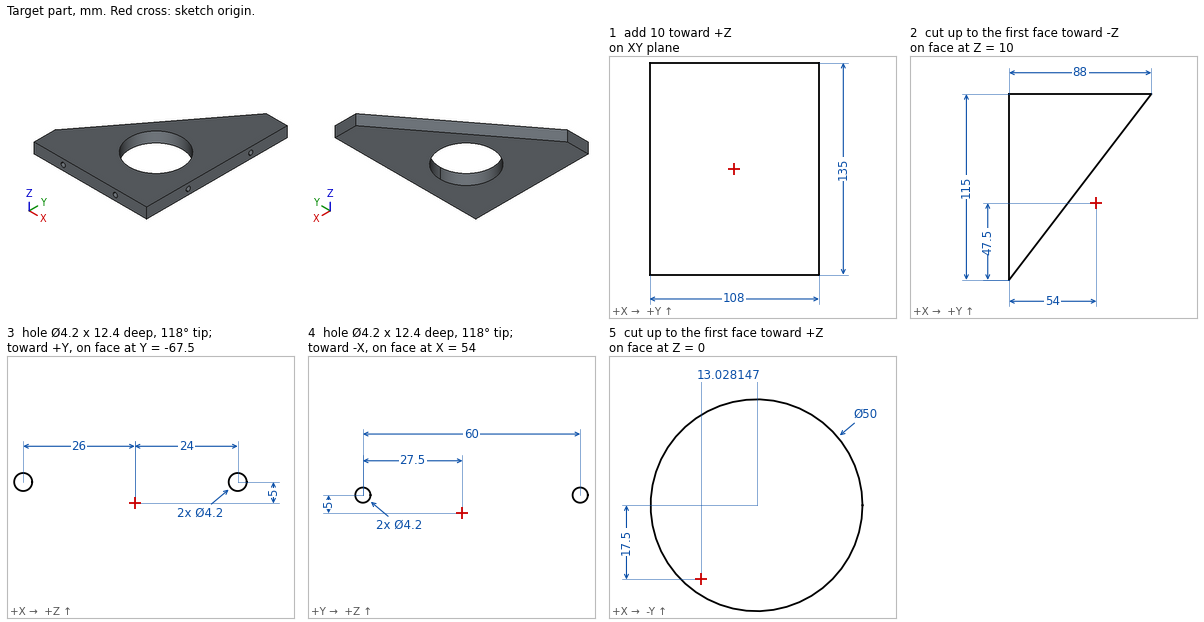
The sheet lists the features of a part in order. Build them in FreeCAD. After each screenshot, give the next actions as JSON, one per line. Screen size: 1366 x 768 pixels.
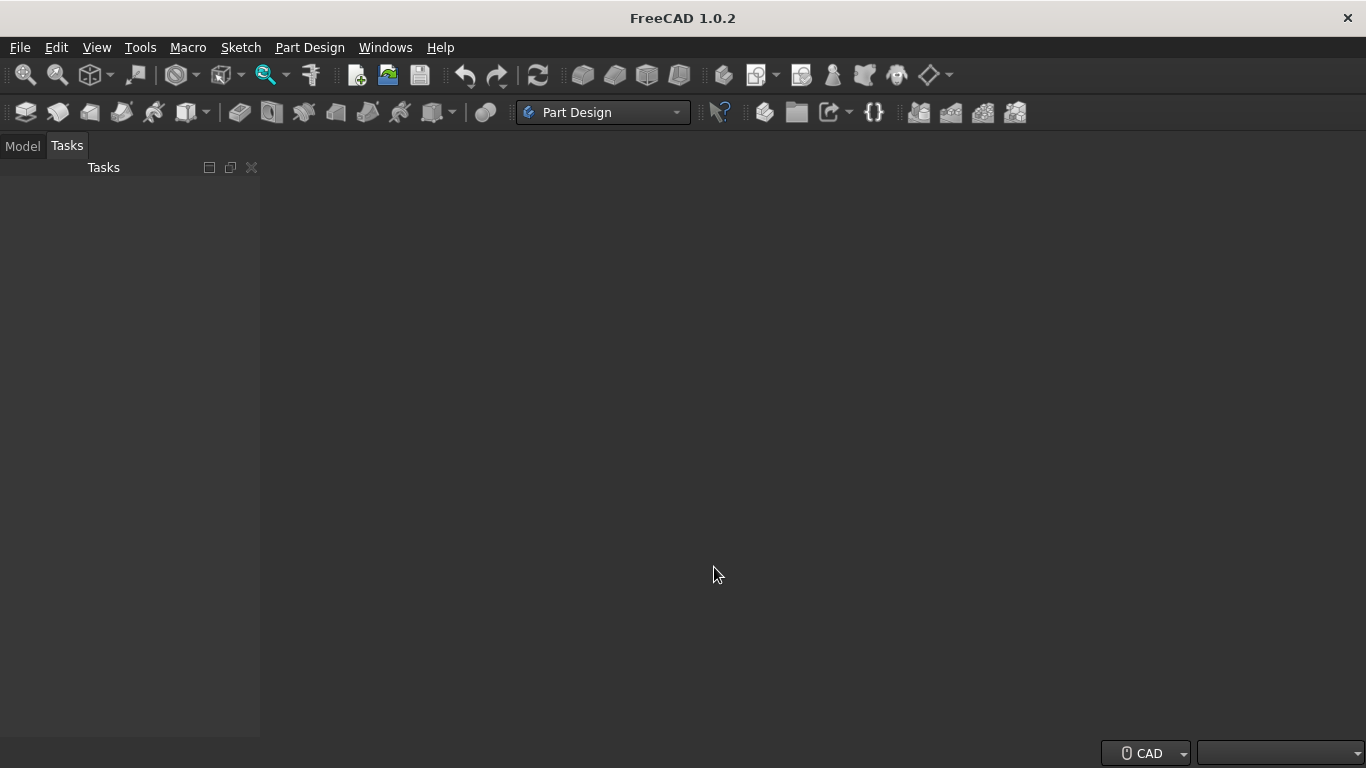
{"action": "key", "text": "ctrl+n"}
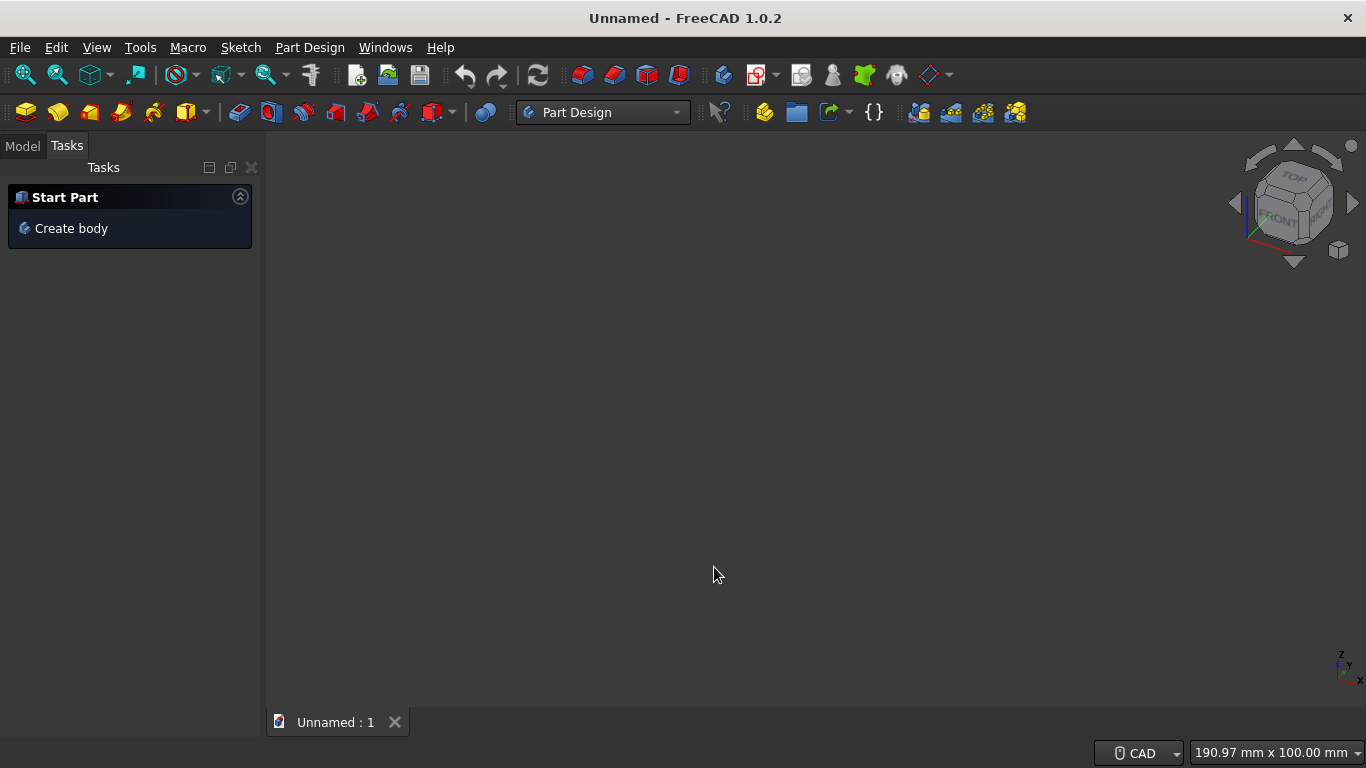
{"action": "left_click", "coordinate": [756, 76]}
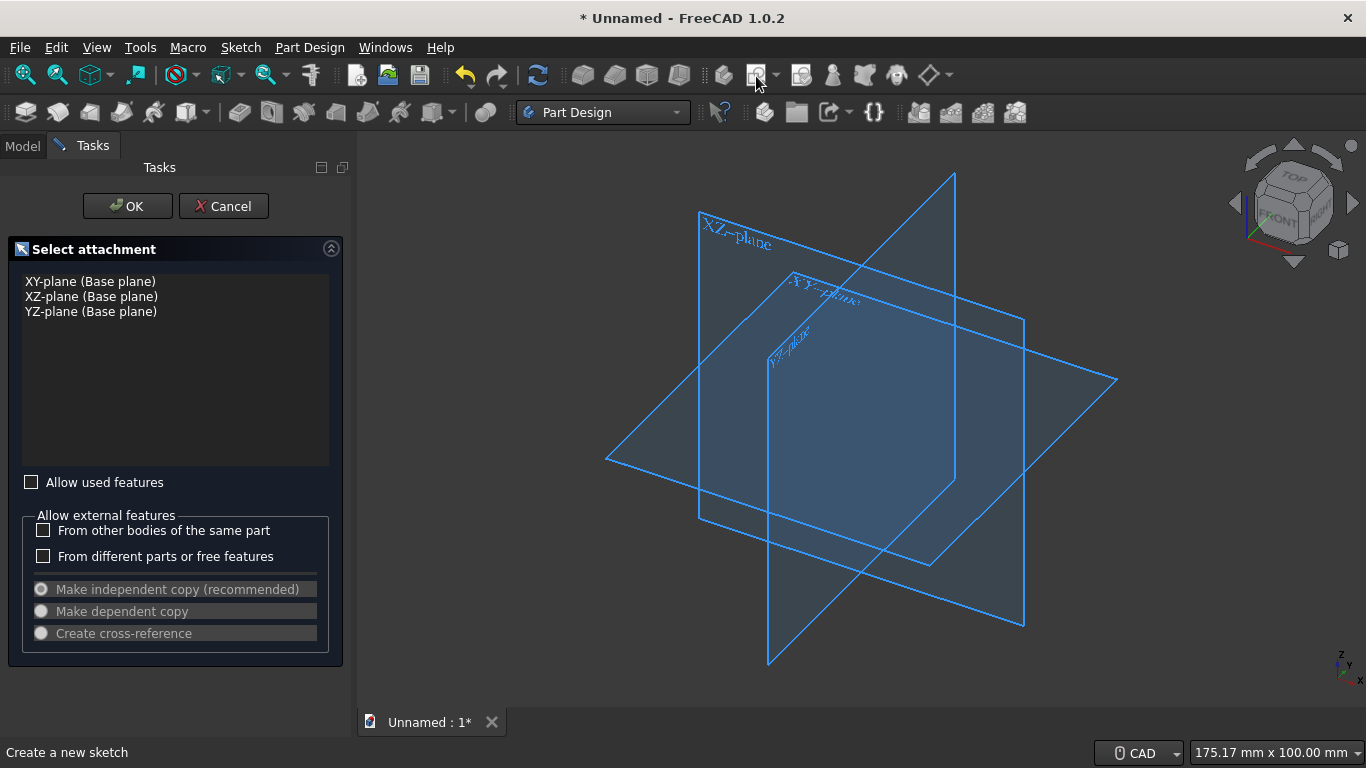
{"action": "left_click", "coordinate": [82, 282]}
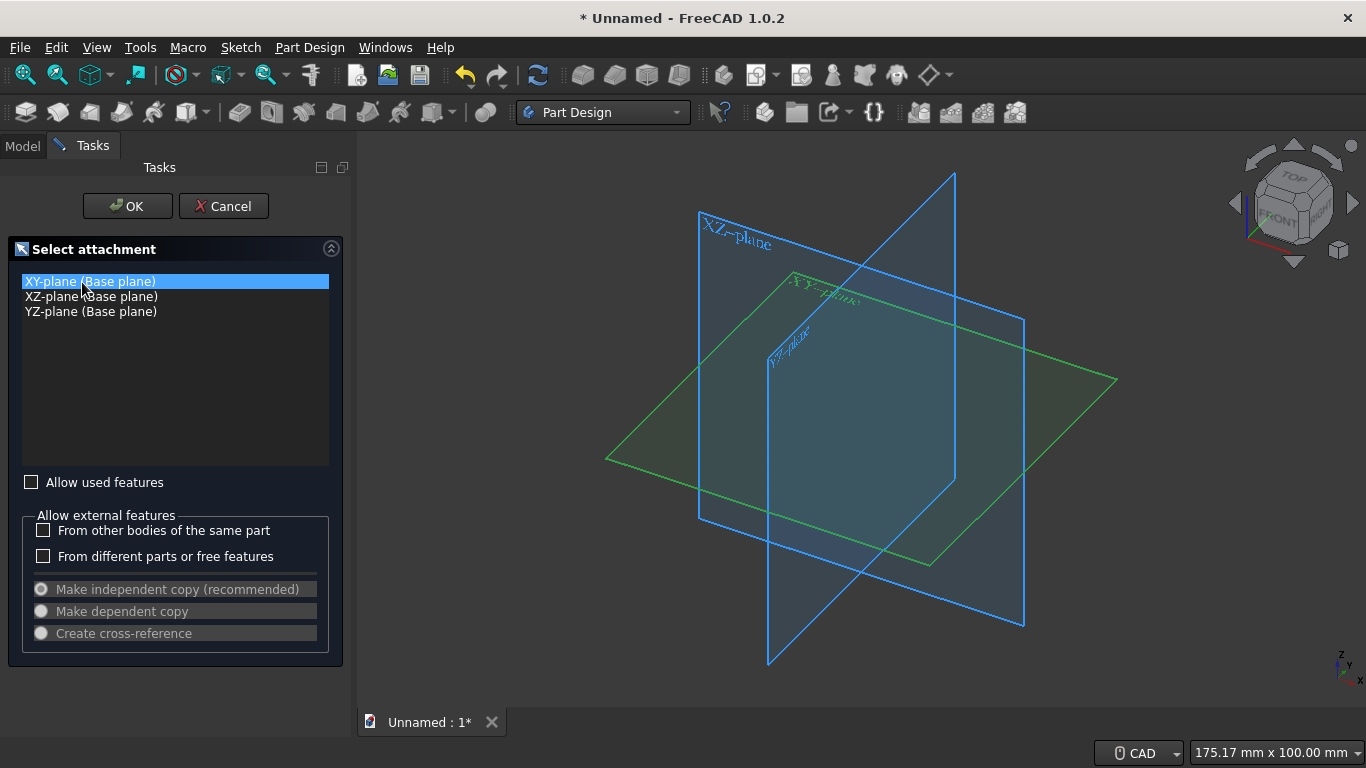
{"action": "left_click", "coordinate": [128, 206]}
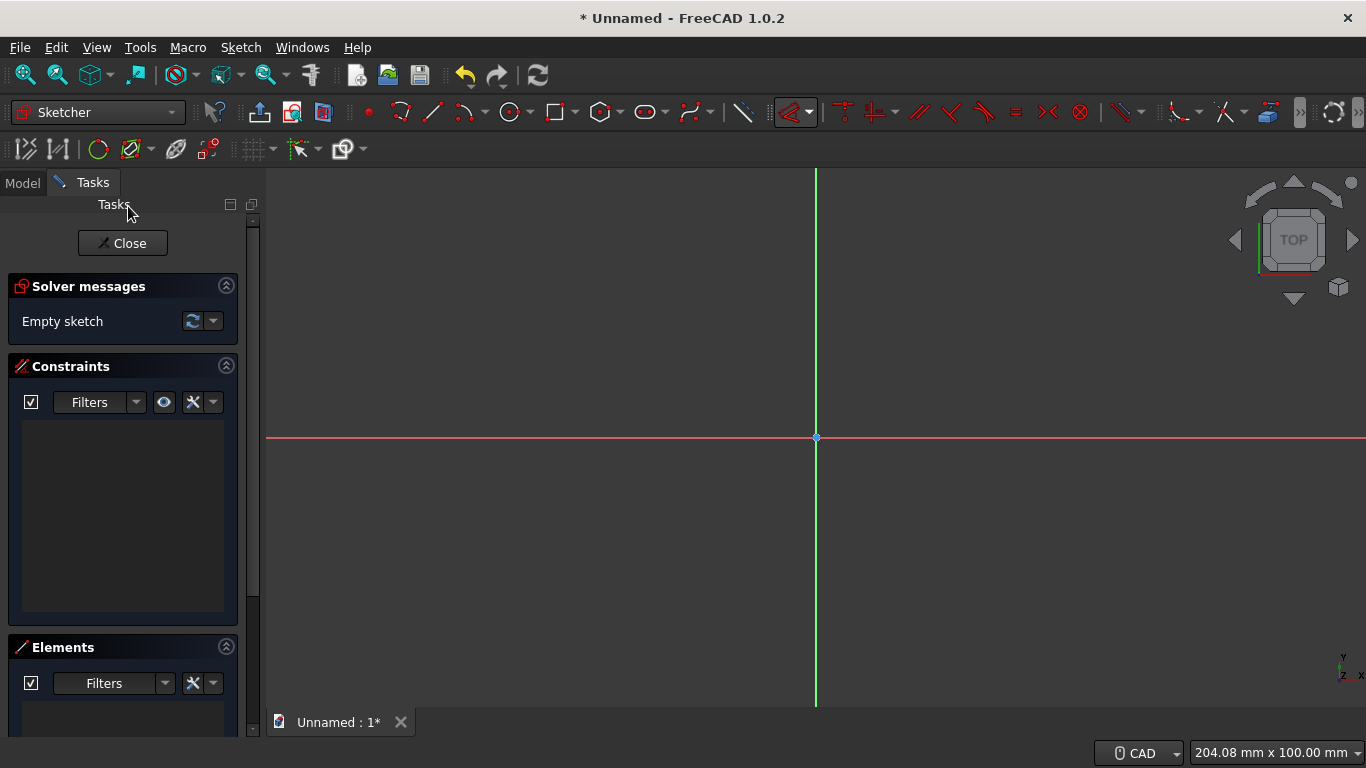
{"action": "scroll", "coordinate": [692, 438], "scroll_direction": "down", "scroll_amount": 4}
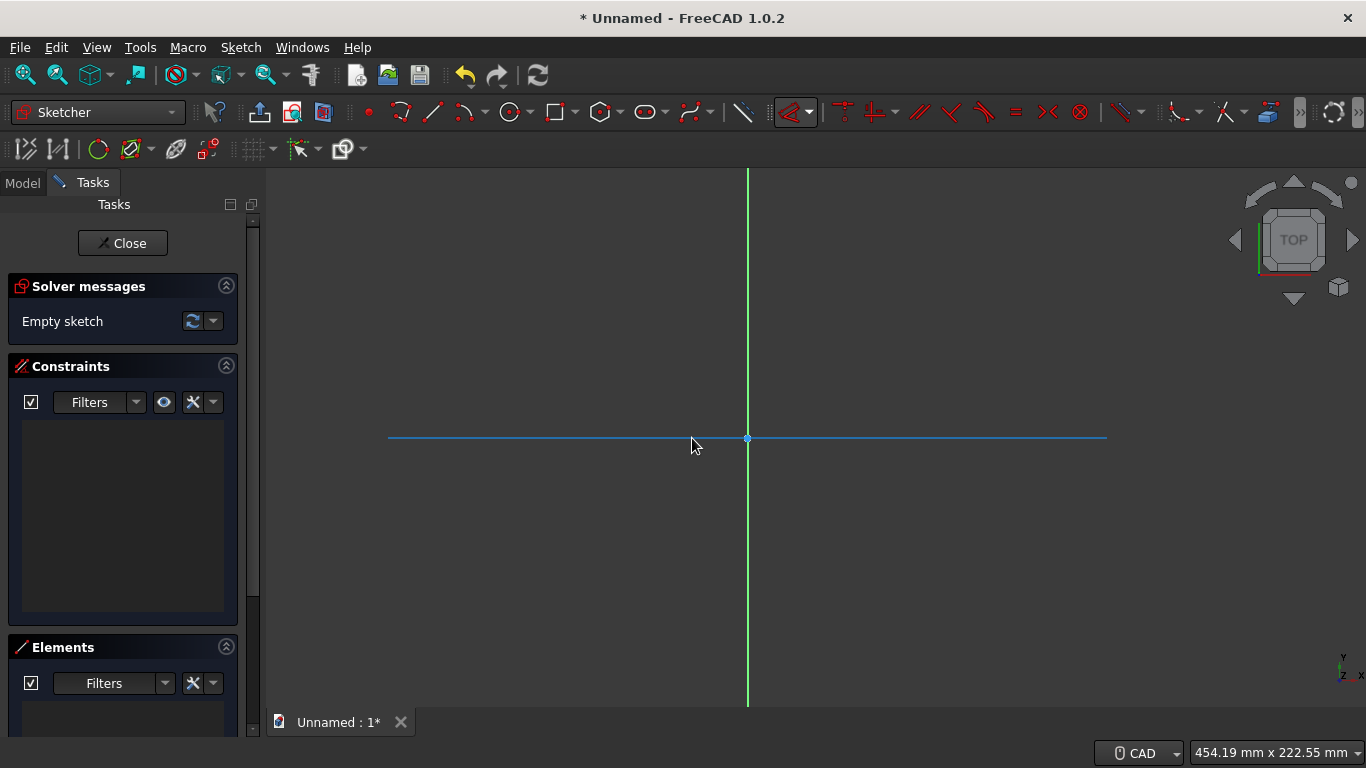
{"action": "key", "text": "g v"}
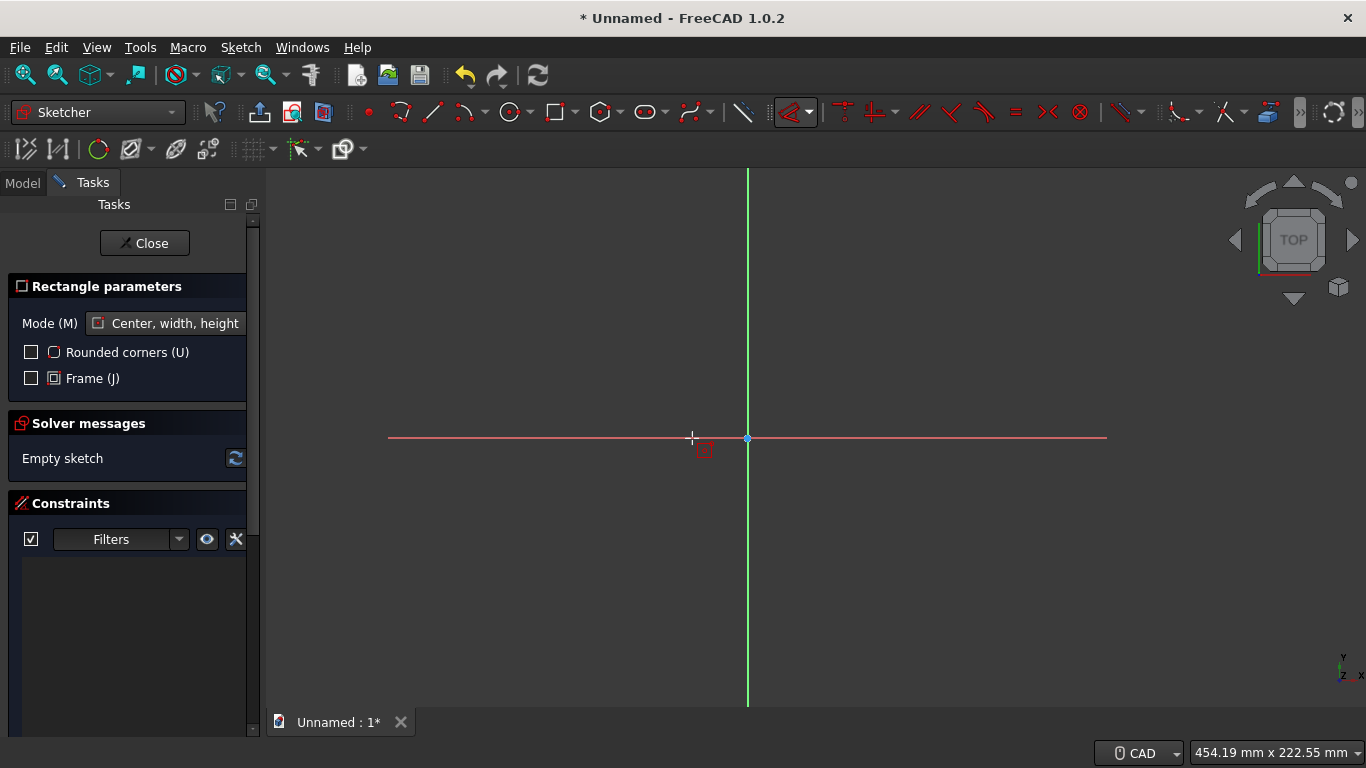
{"action": "left_click", "coordinate": [748, 438]}
{"action": "mouse_move", "coordinate": [879, 275]}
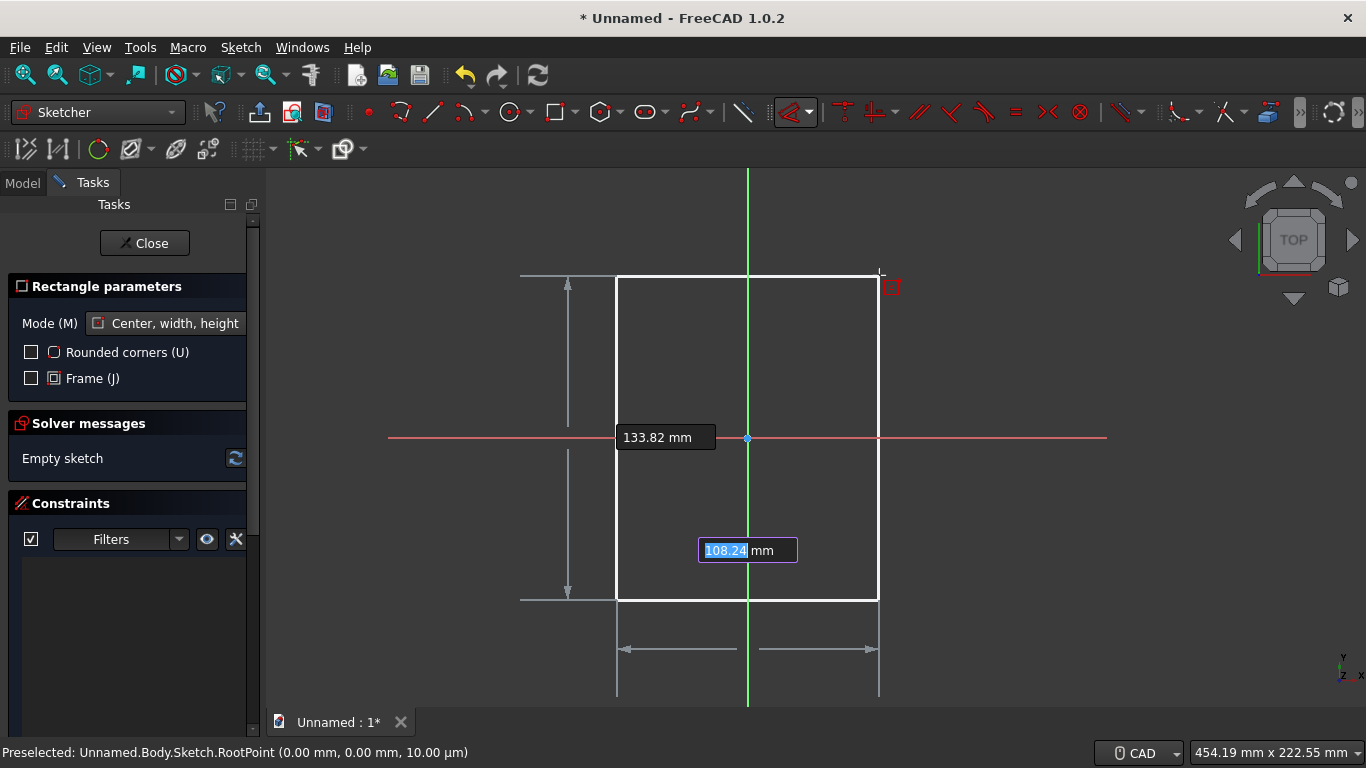
{"action": "type", "text": "108"}
{"action": "key", "text": "Tab"}
{"action": "type", "text": "135"}
{"action": "key", "text": "Return"}
{"action": "key", "text": "Escape"}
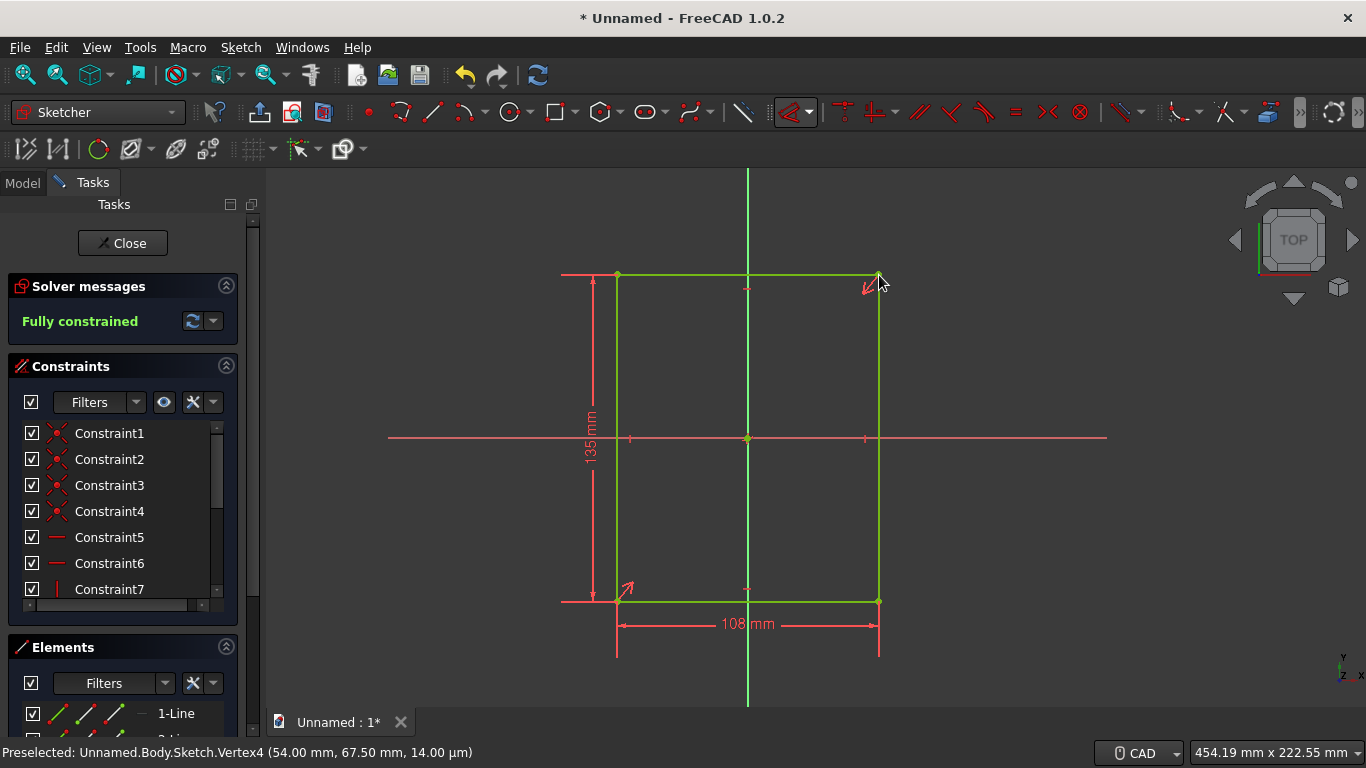
{"action": "left_click", "coordinate": [123, 243]}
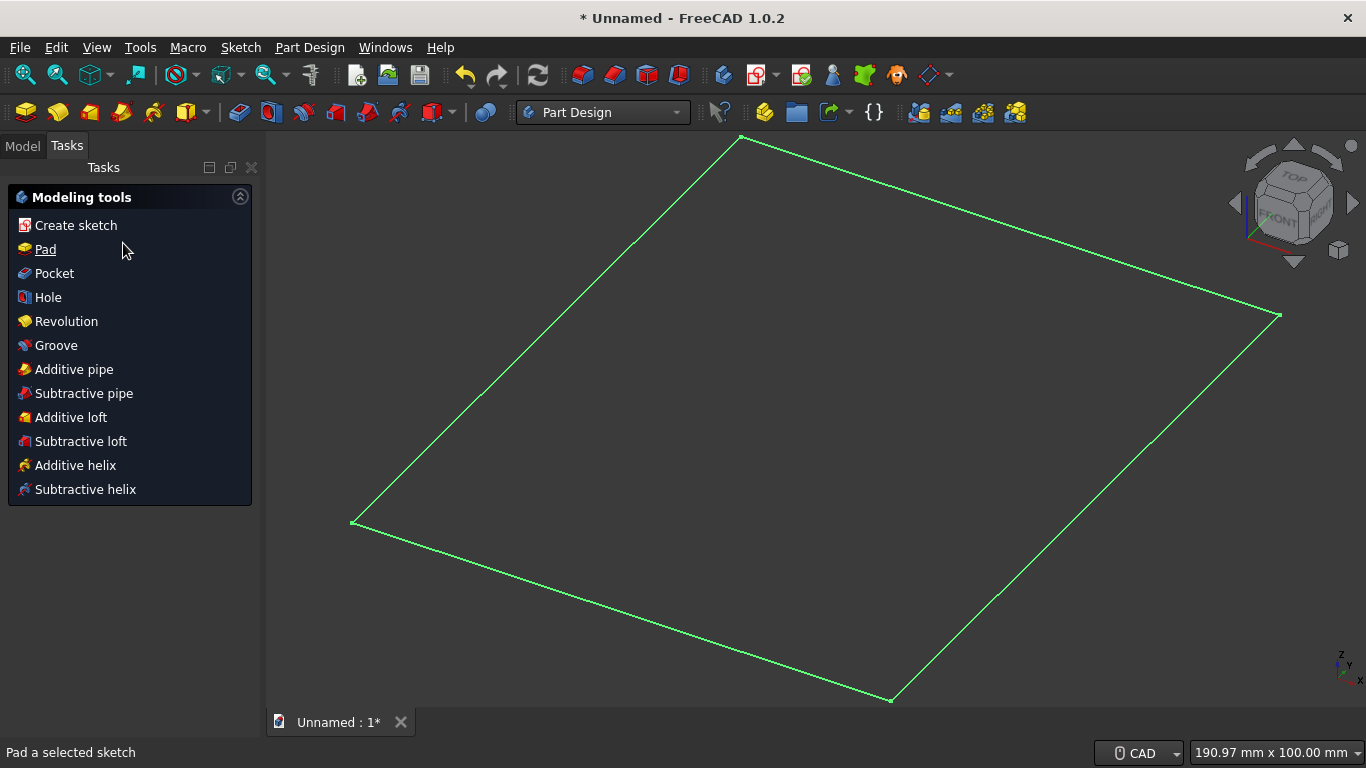
{"action": "left_click", "coordinate": [26, 112]}